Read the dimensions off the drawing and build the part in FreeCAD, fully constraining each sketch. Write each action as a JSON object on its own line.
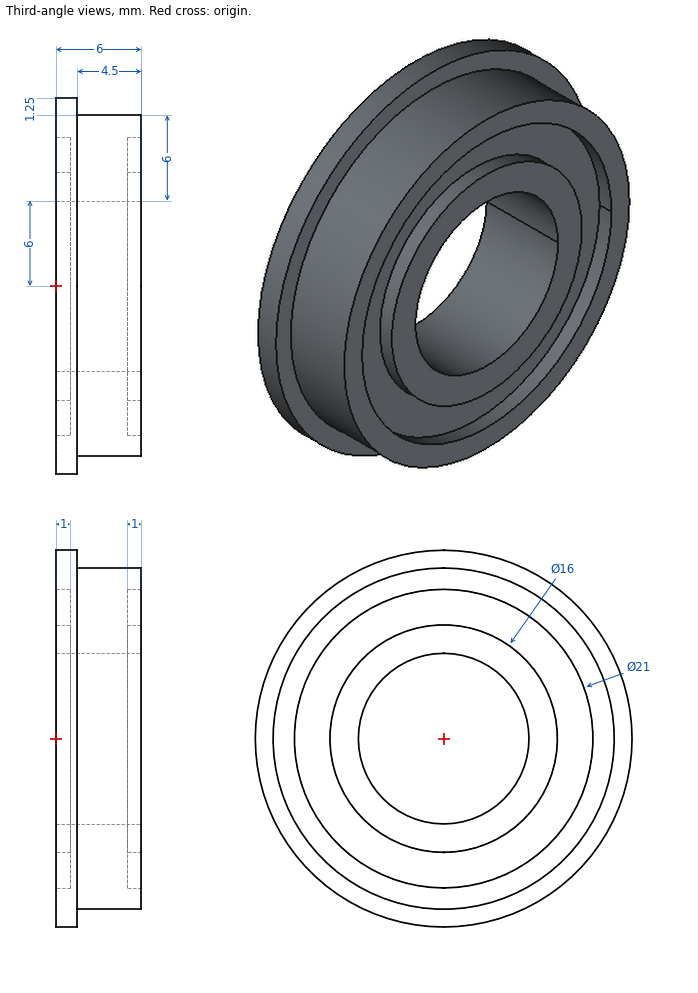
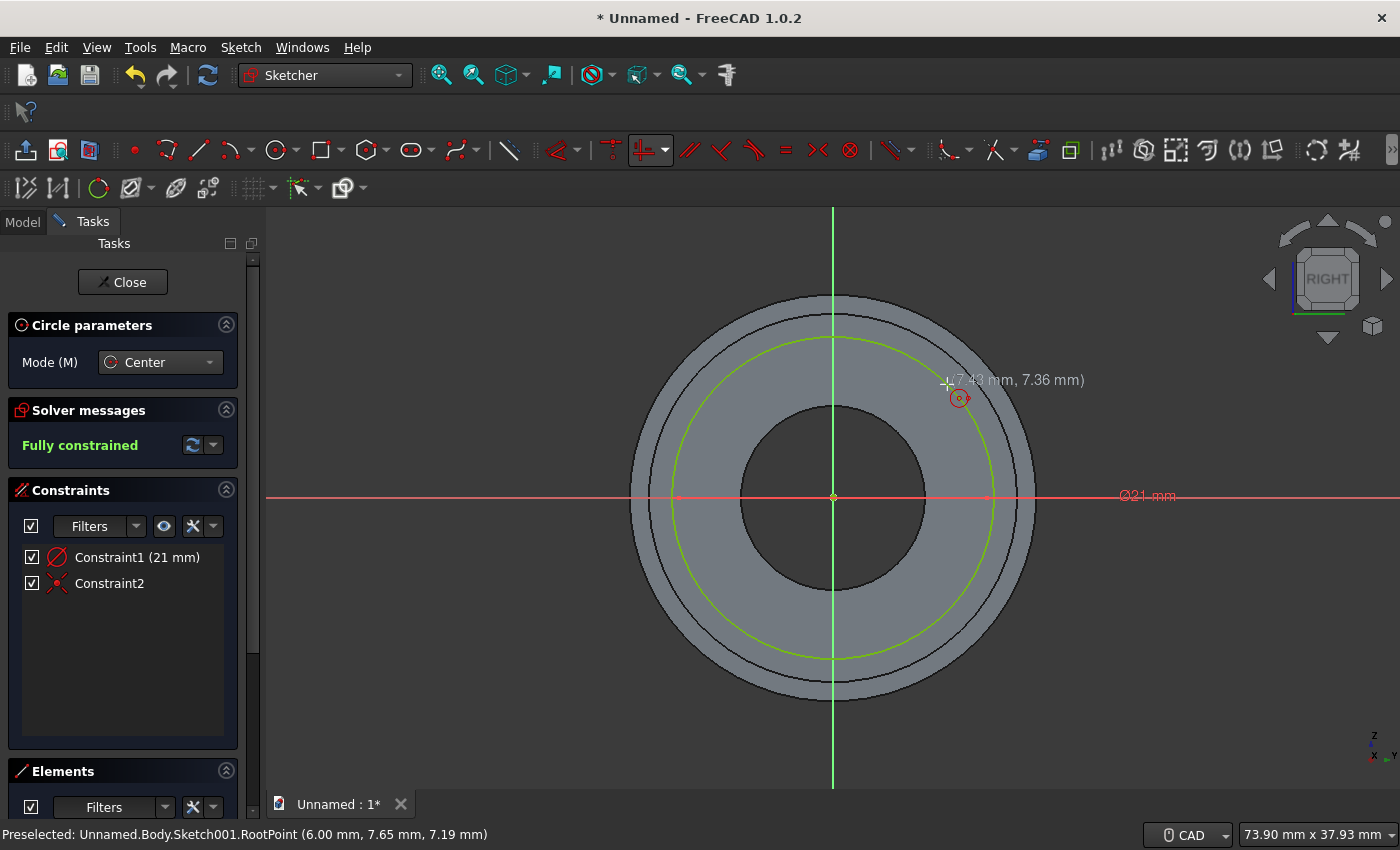
{"action": "left_click", "coordinate": [833, 498]}
{"action": "mouse_move", "coordinate": [920, 411]}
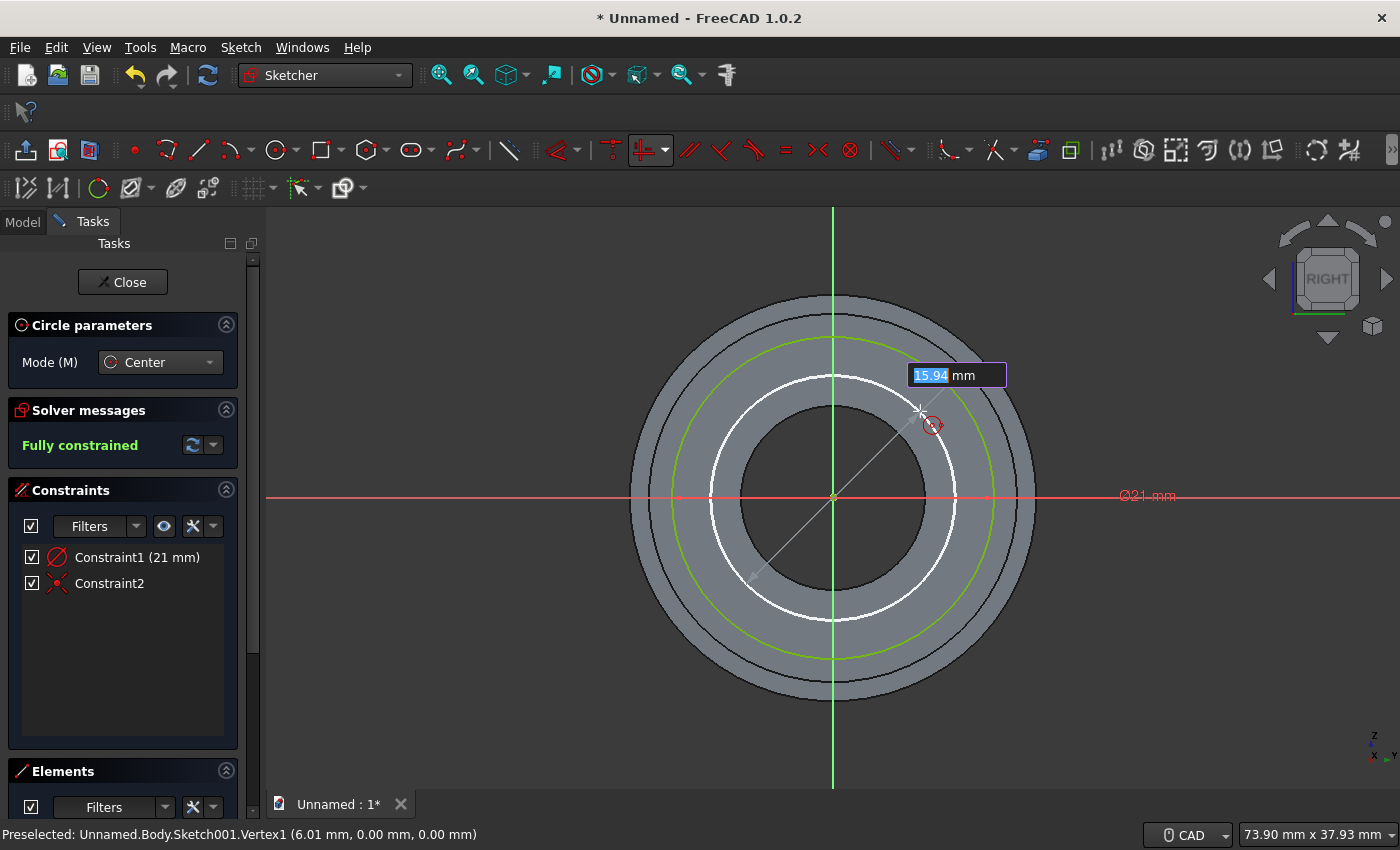
{"action": "type", "text": "16"}
{"action": "key", "text": "Return"}
{"action": "key", "text": "Escape"}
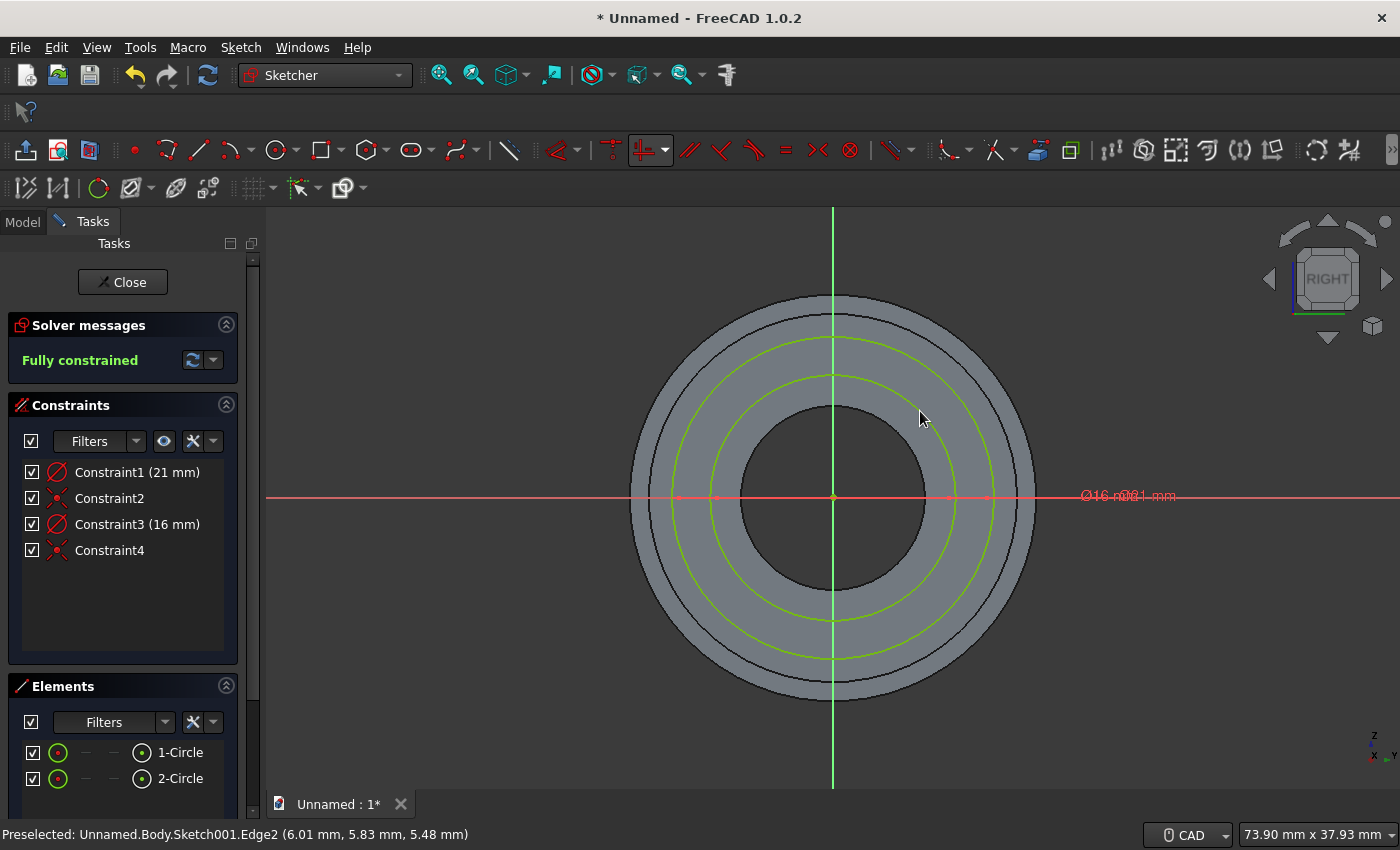
{"action": "left_click", "coordinate": [123, 282]}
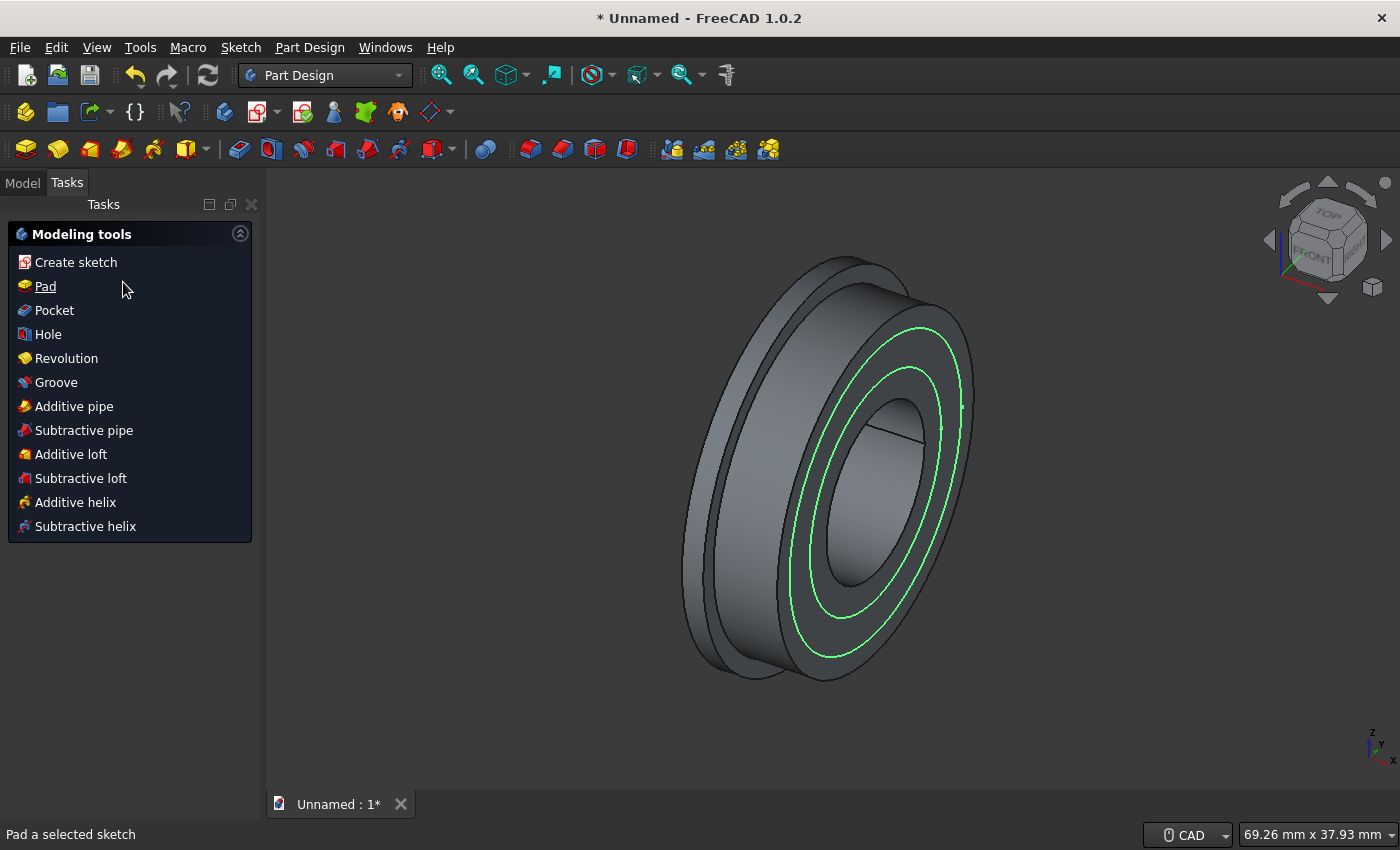
{"action": "left_click", "coordinate": [240, 150]}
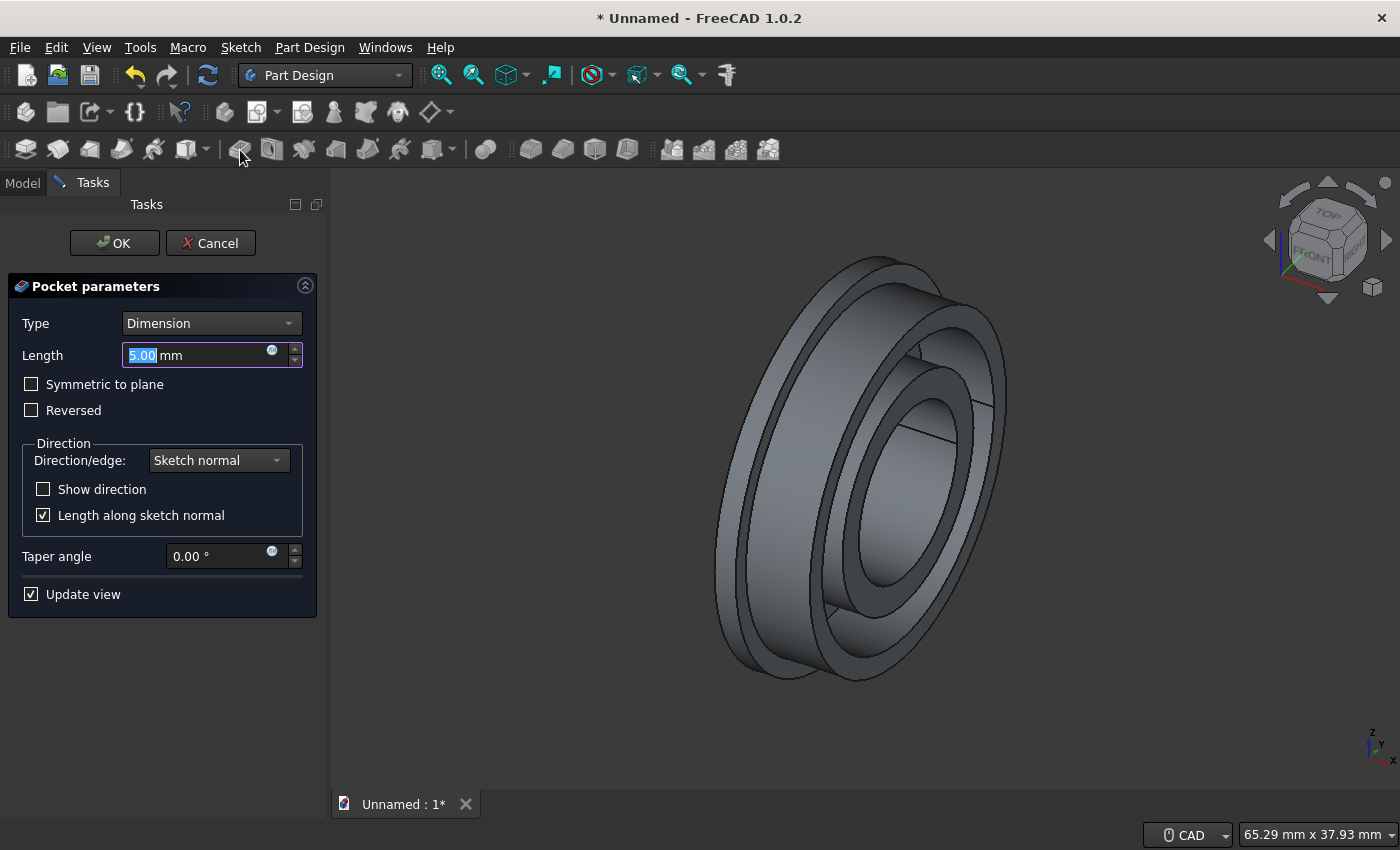
{"action": "type", "text": "1"}
{"action": "key", "text": "Tab"}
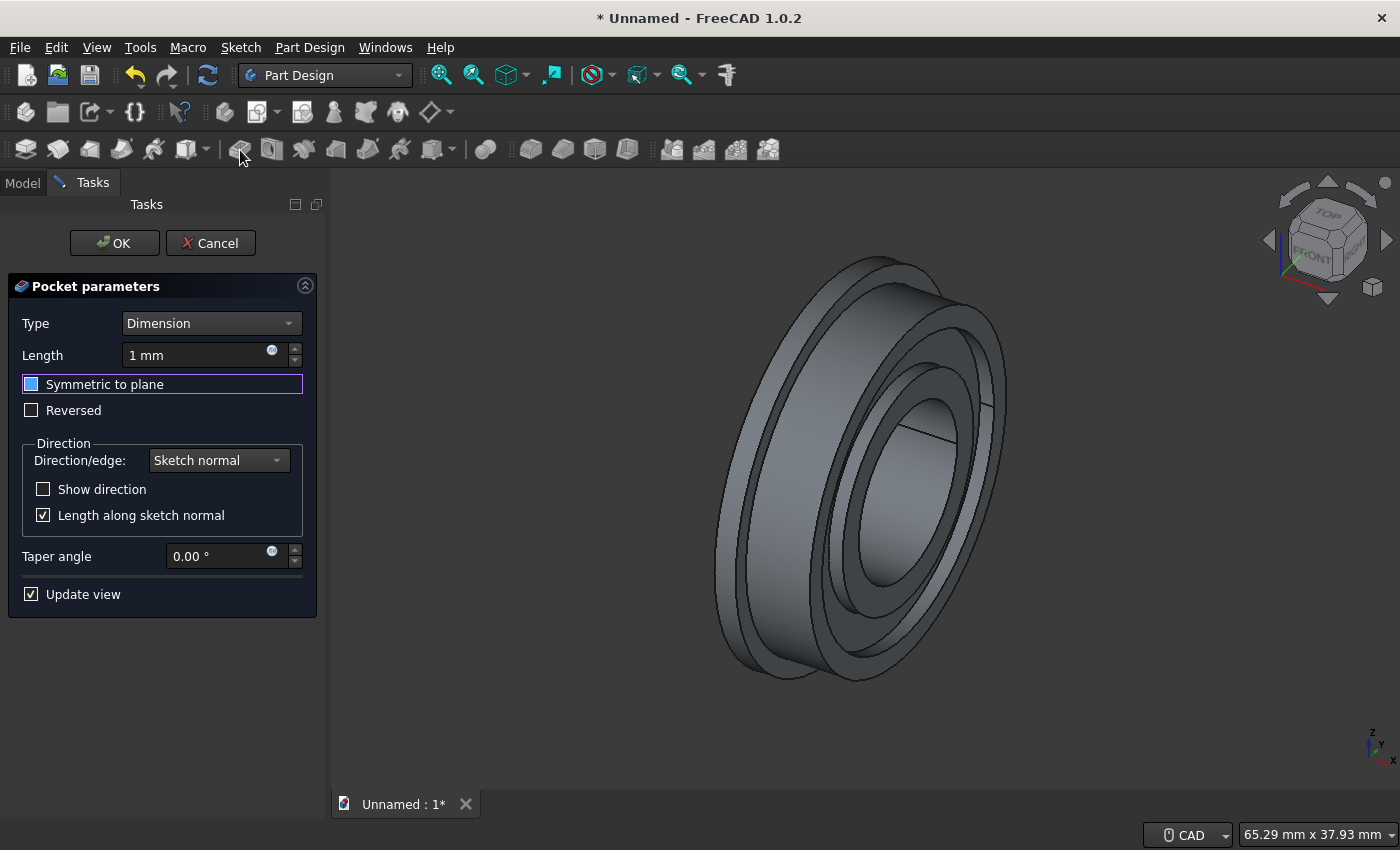
{"action": "left_click", "coordinate": [115, 243]}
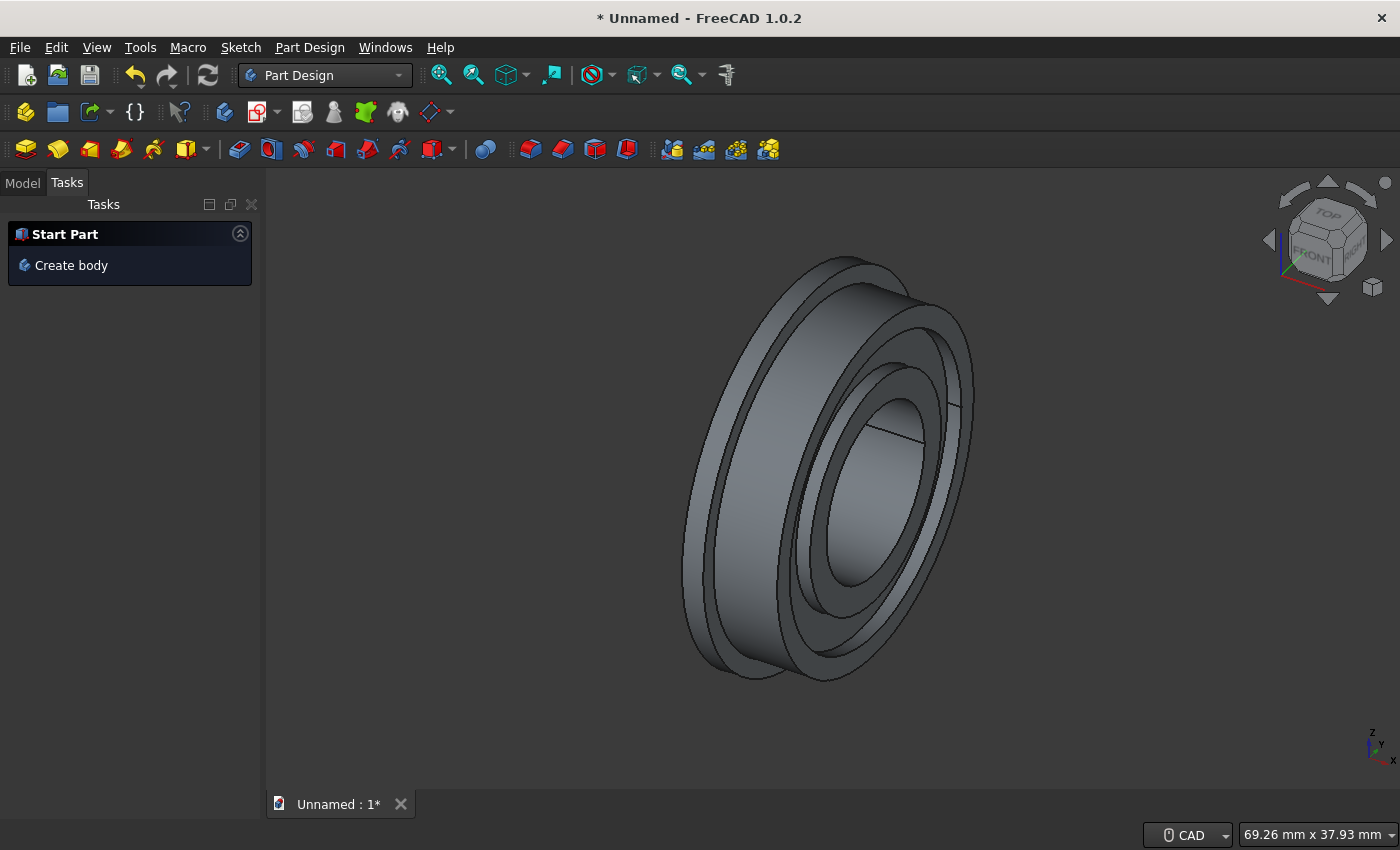
{"action": "left_click", "coordinate": [23, 182]}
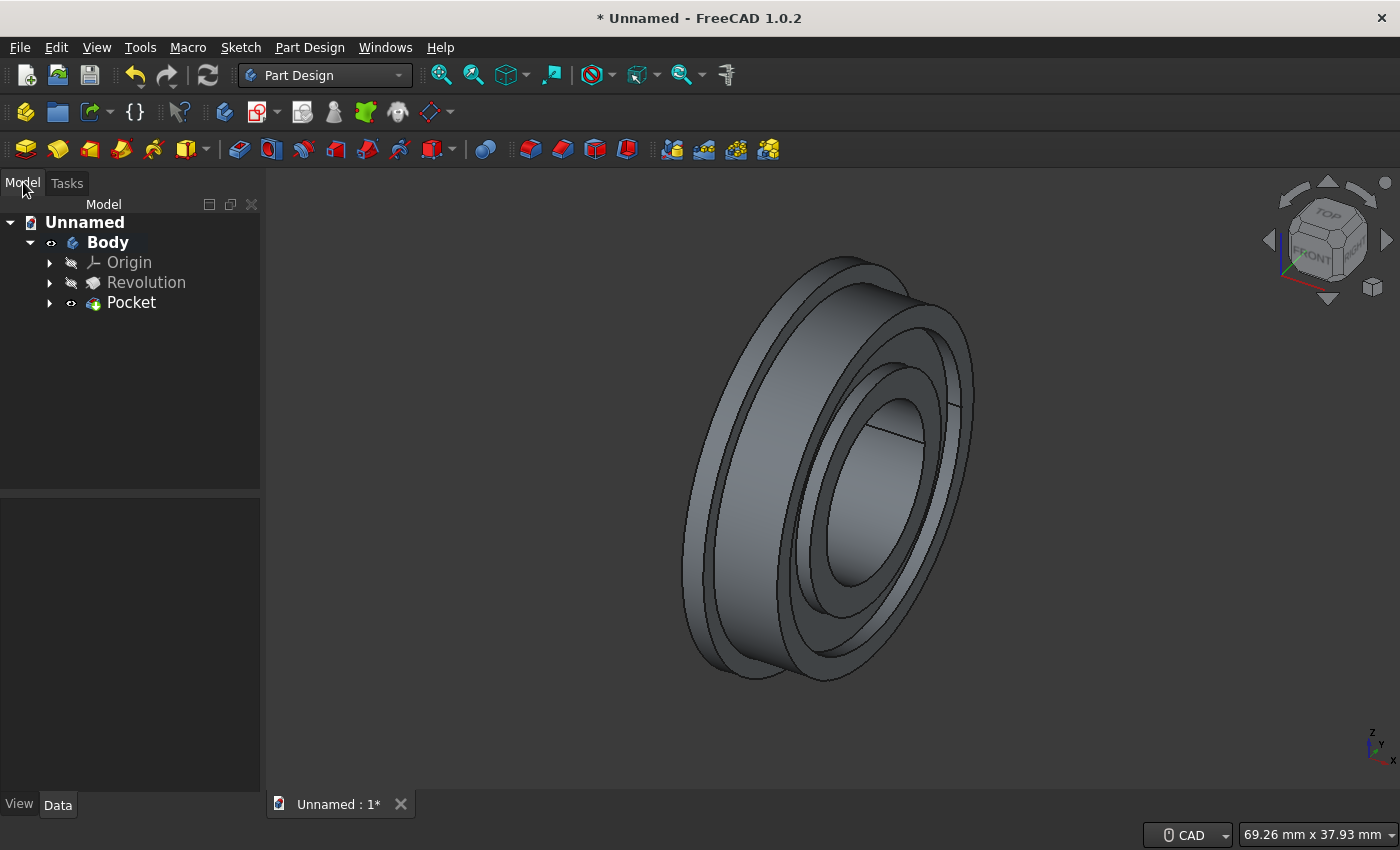
{"action": "left_click", "coordinate": [50, 263]}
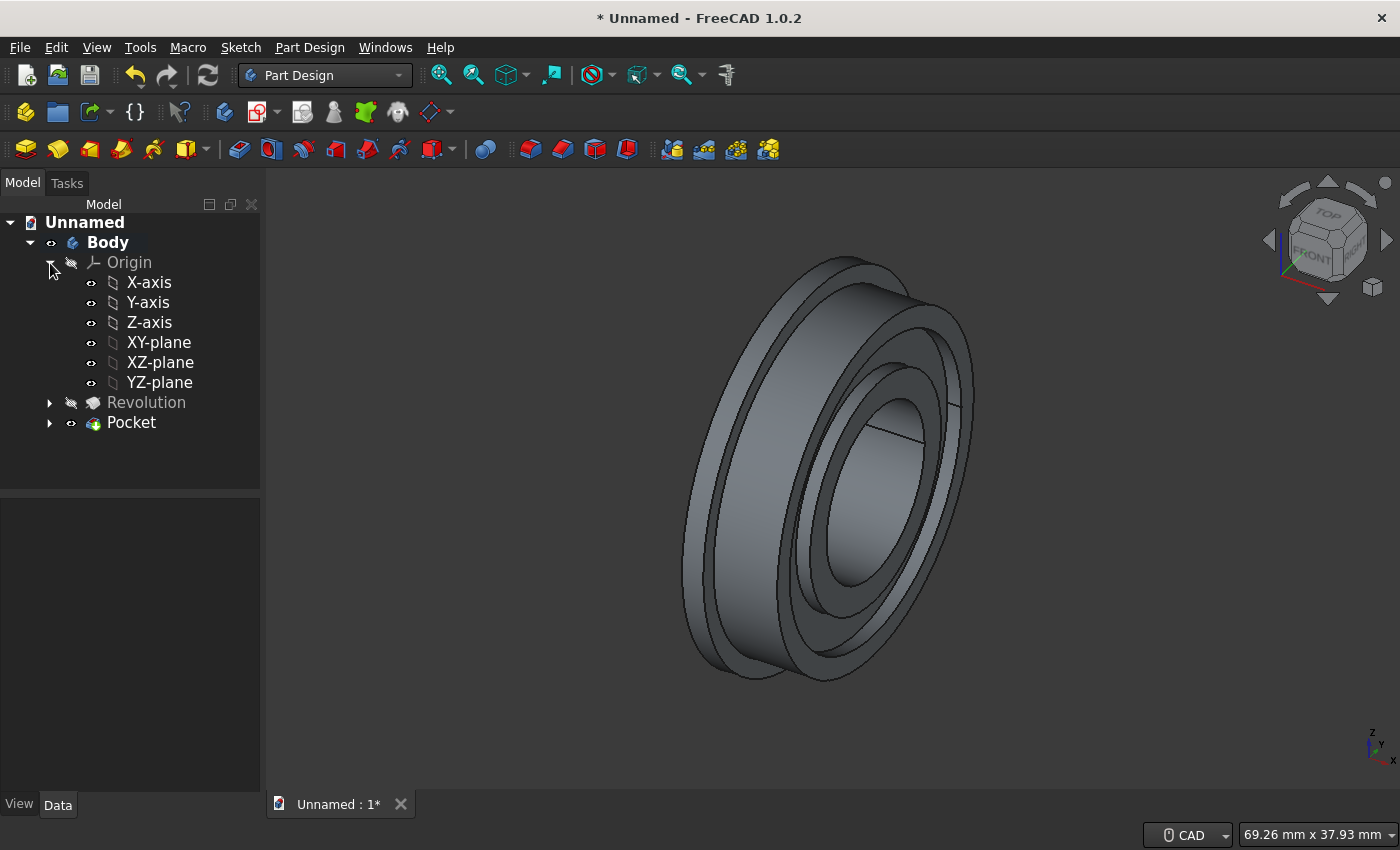
{"action": "left_click", "coordinate": [136, 383]}